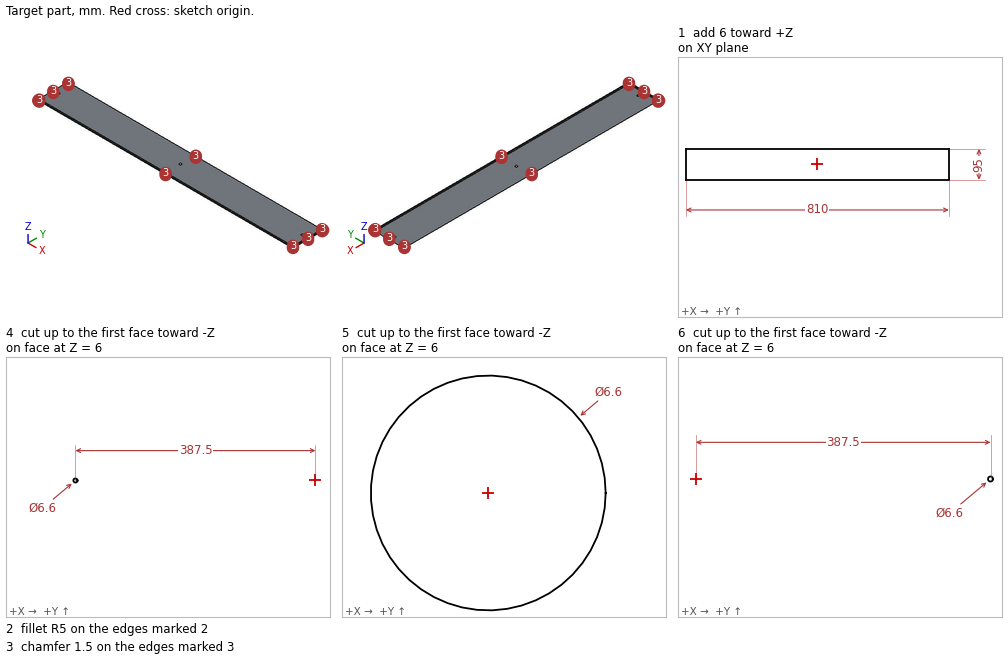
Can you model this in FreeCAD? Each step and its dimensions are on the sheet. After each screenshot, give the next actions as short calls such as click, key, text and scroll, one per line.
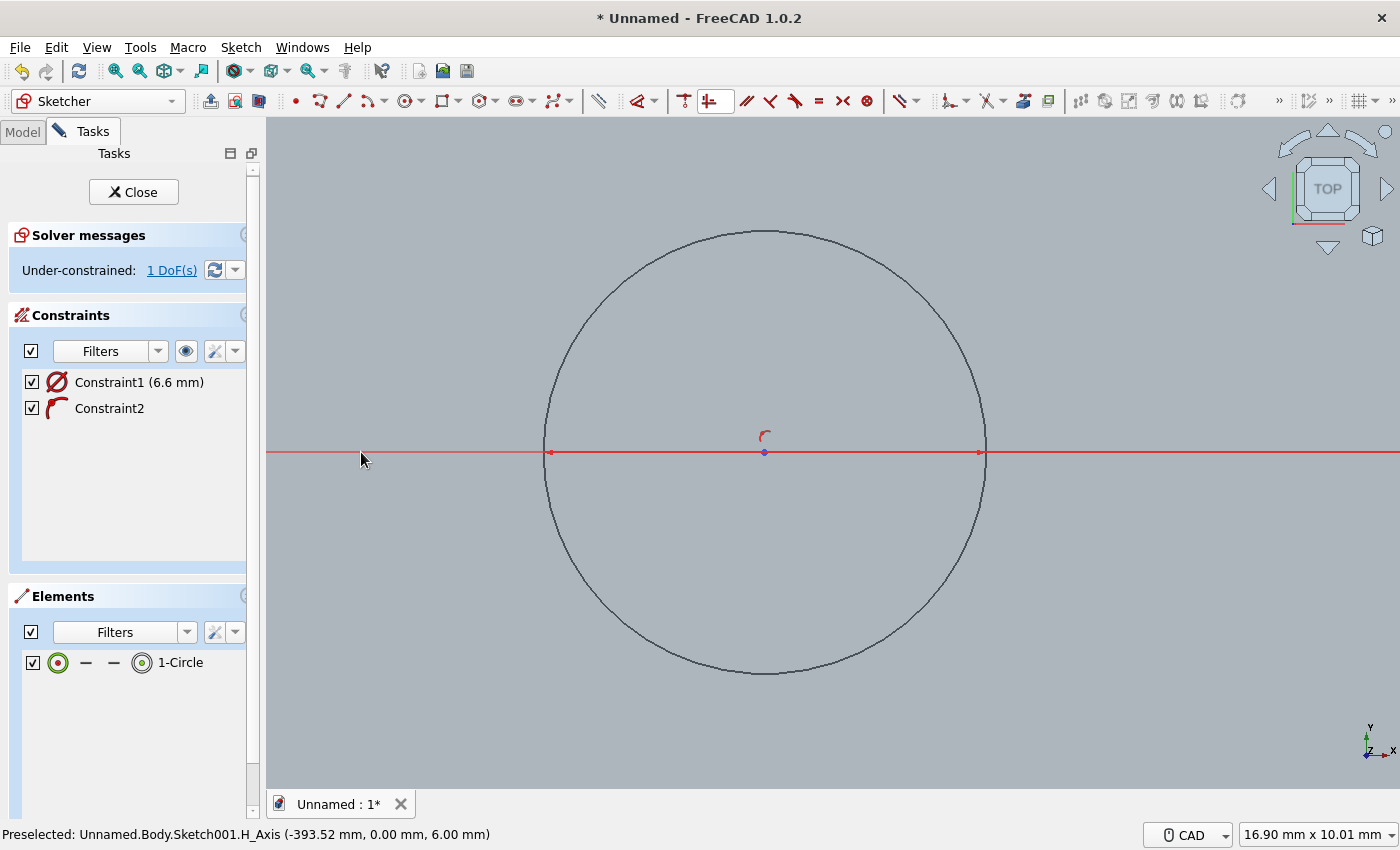
click(638, 102)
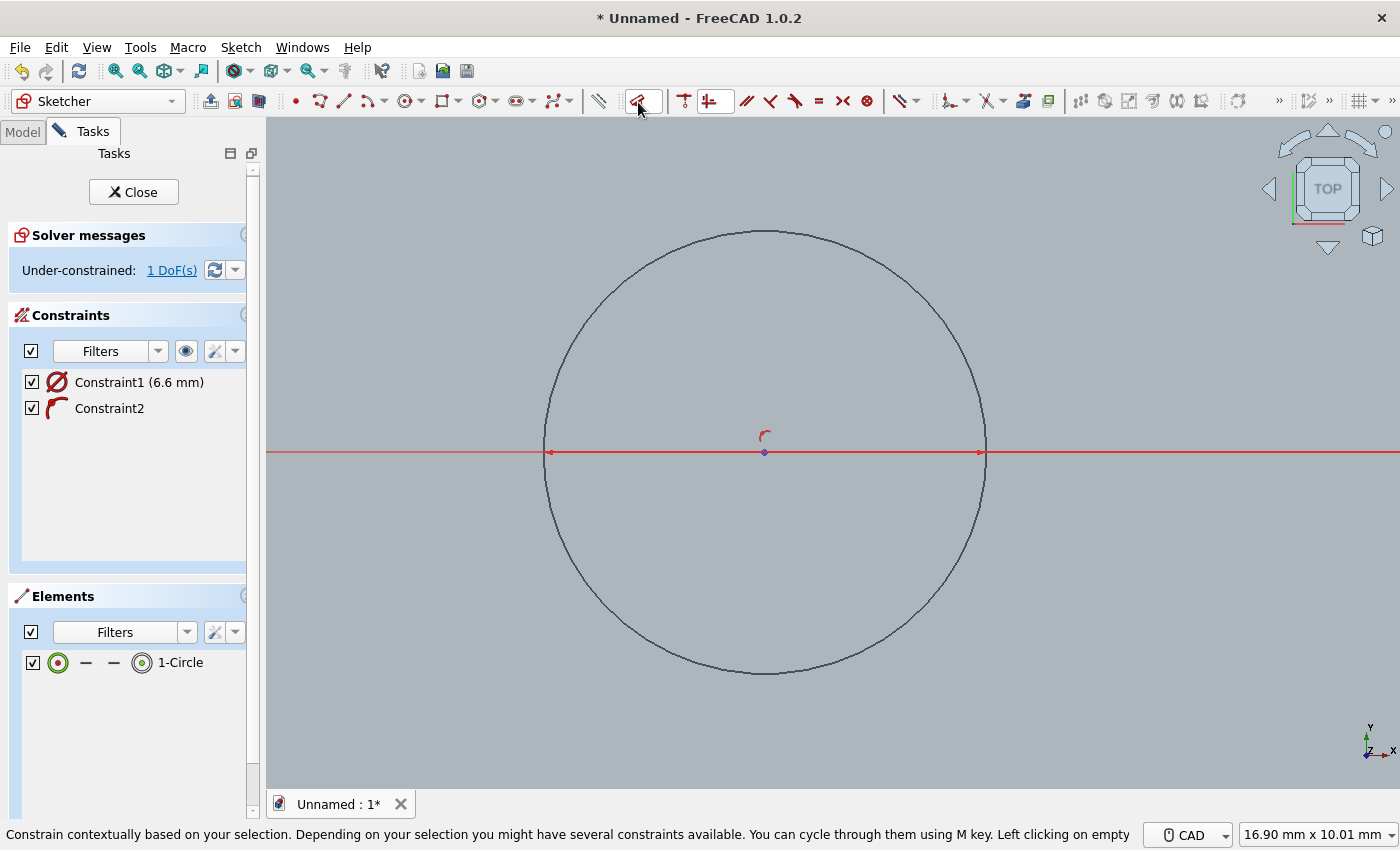
click(765, 452)
click(1000, 486)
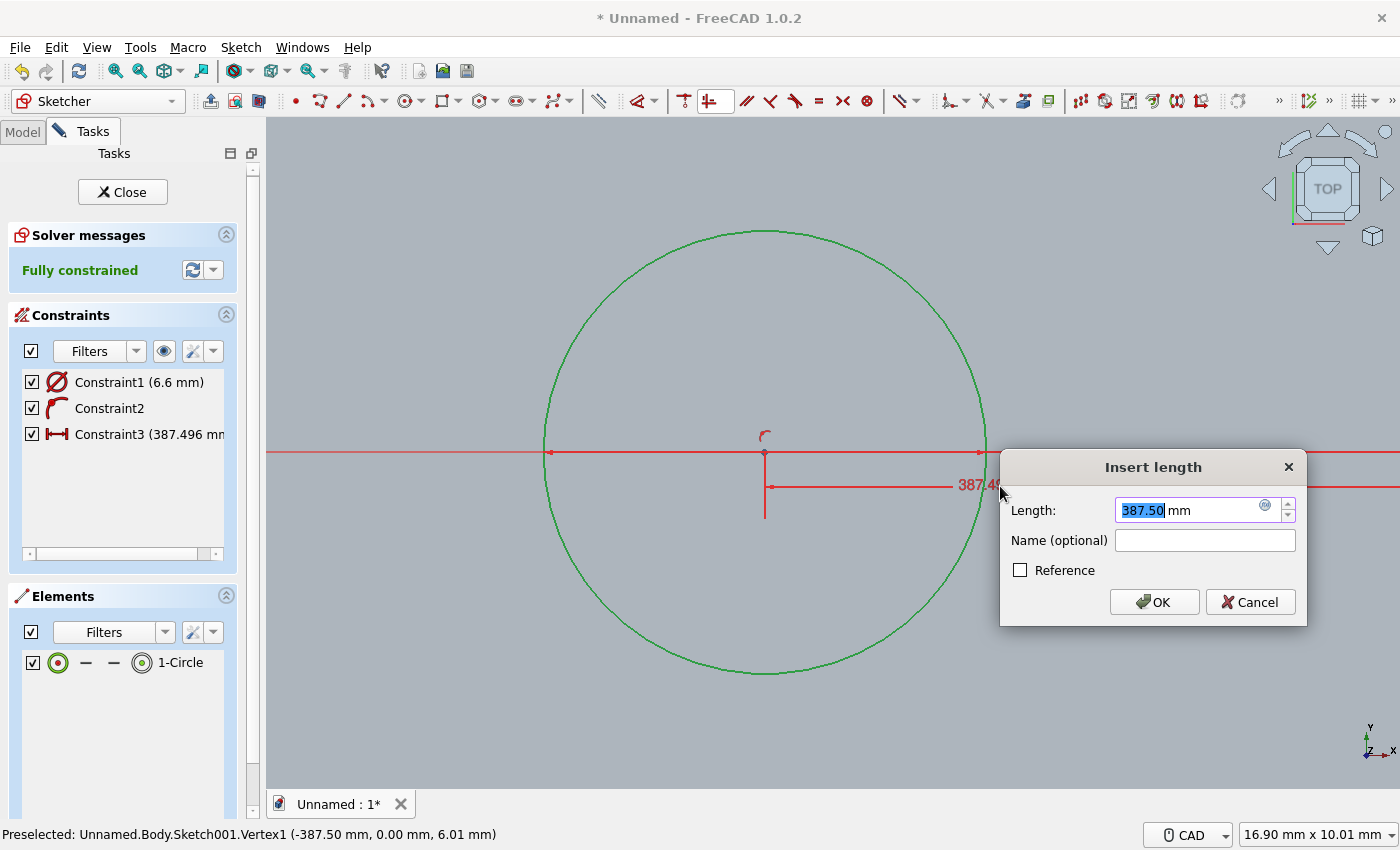
text(387.5)
key(Return)
key(Escape)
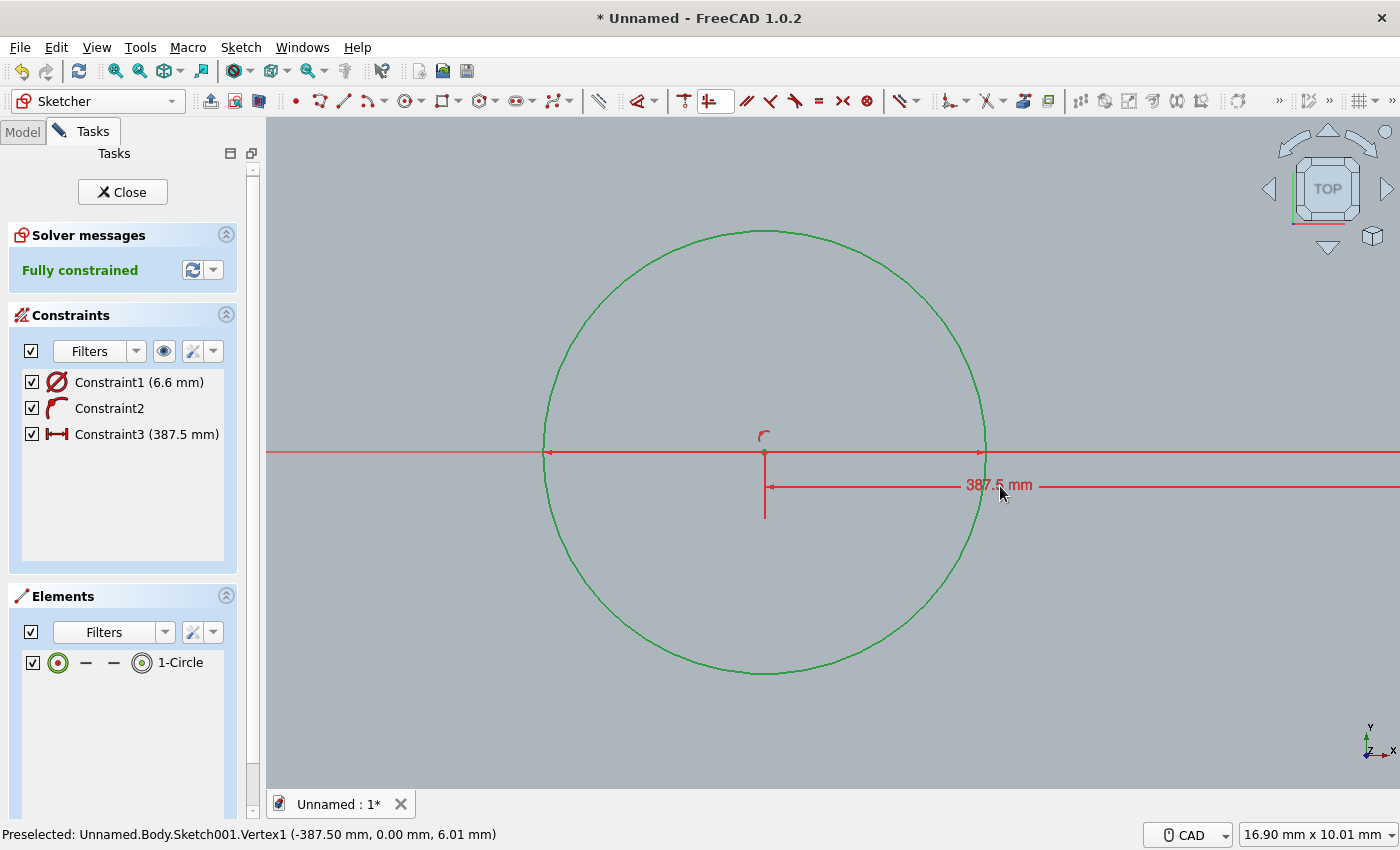
click(123, 192)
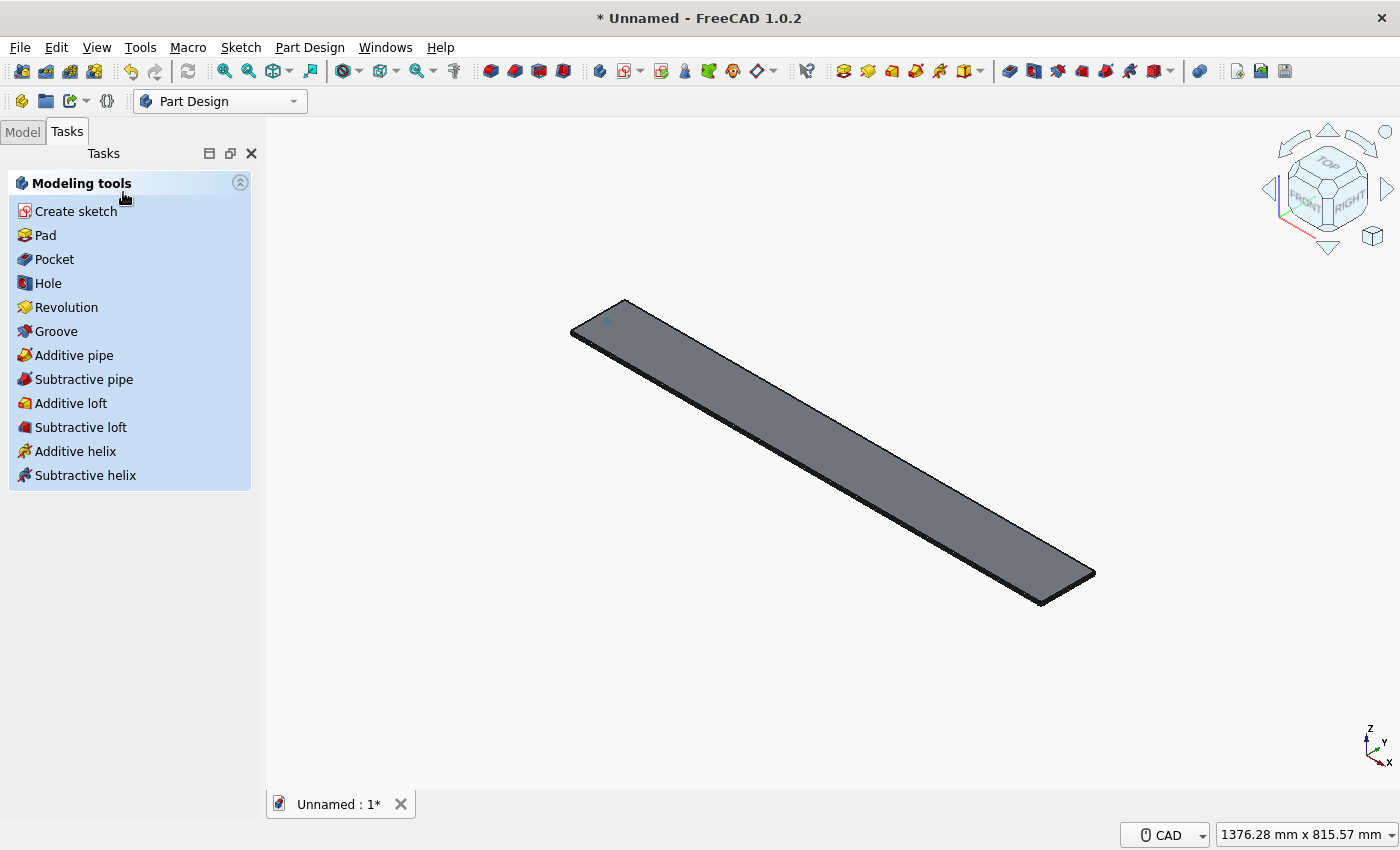
click(1010, 72)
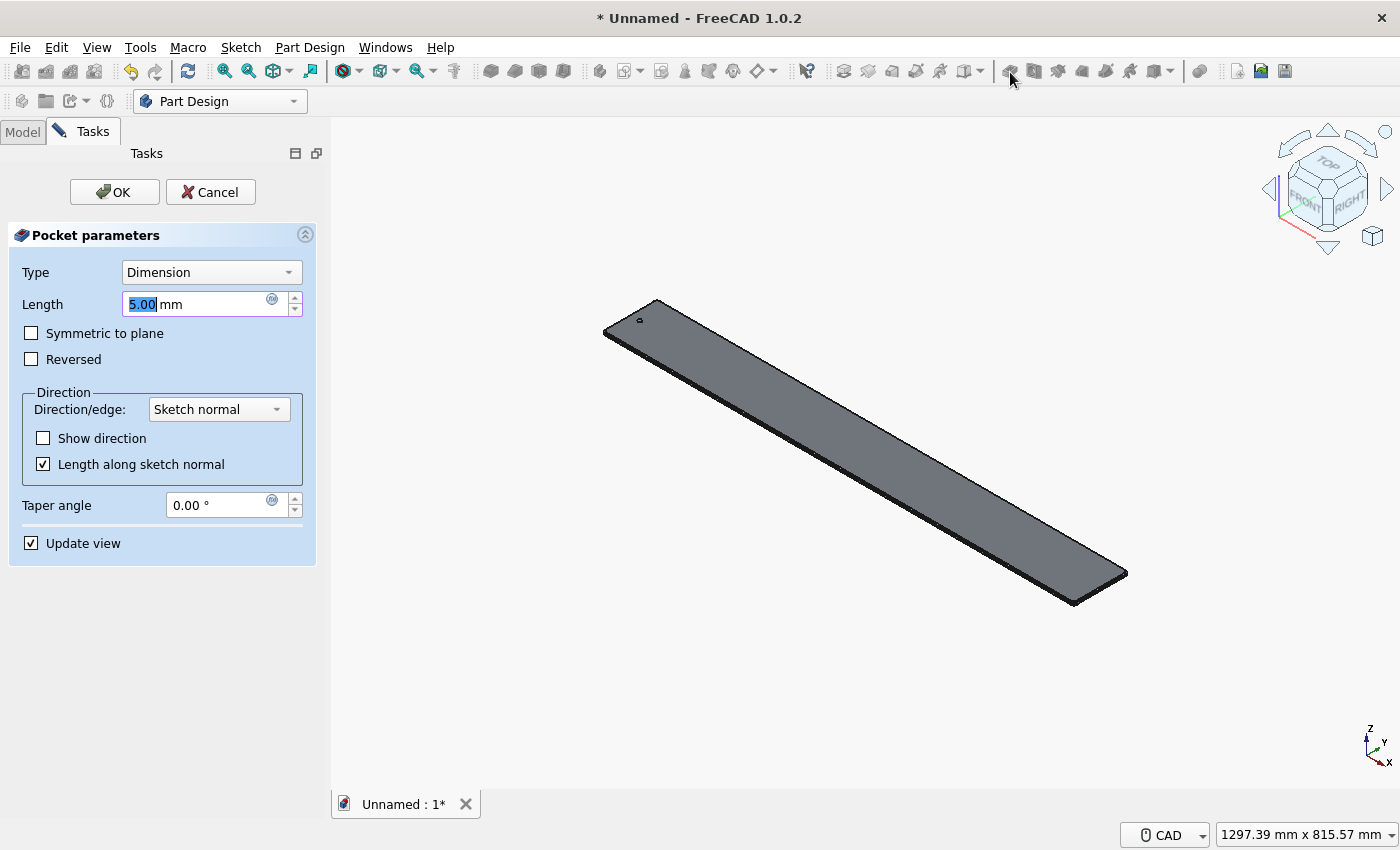
click(212, 272)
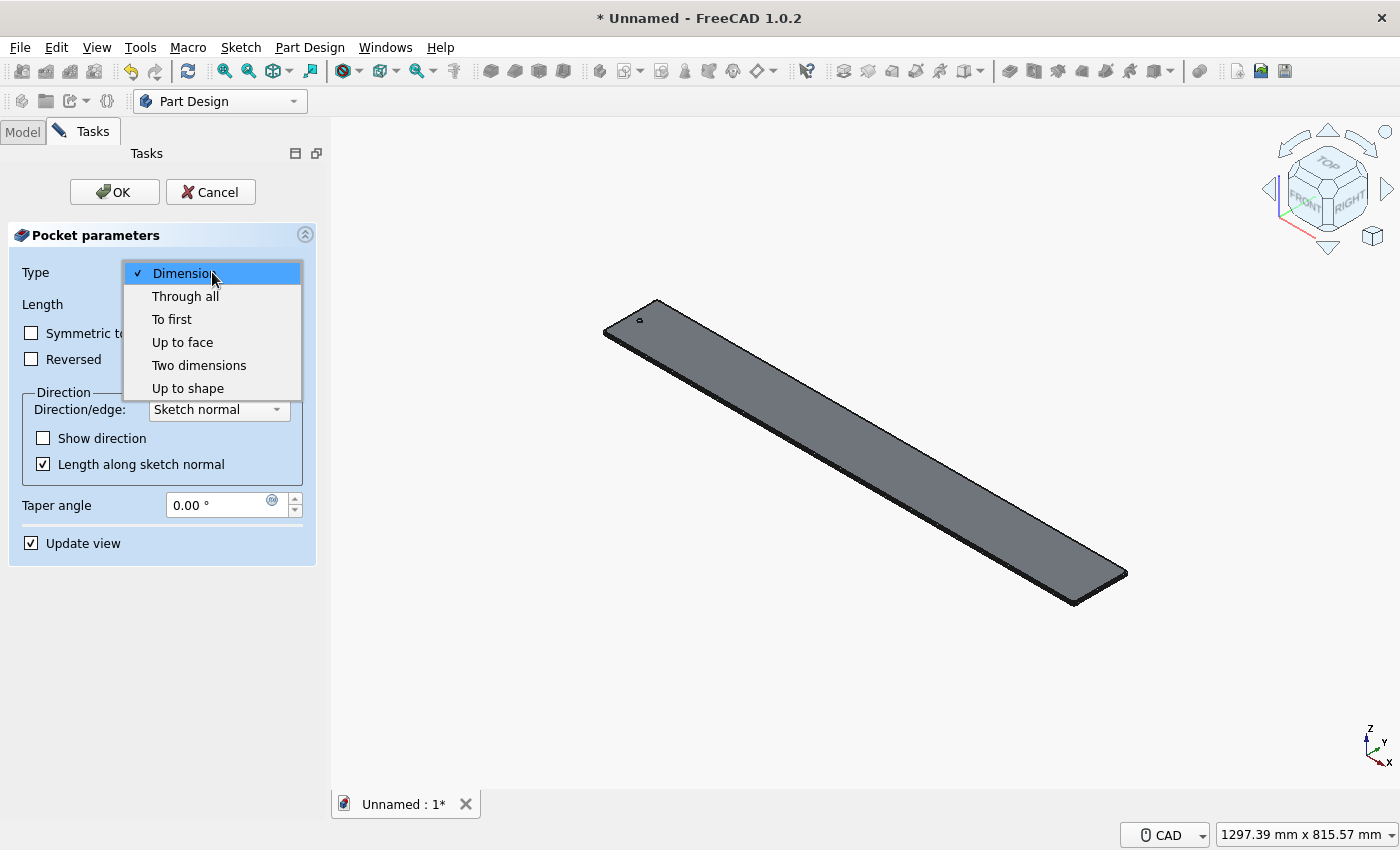
click(212, 320)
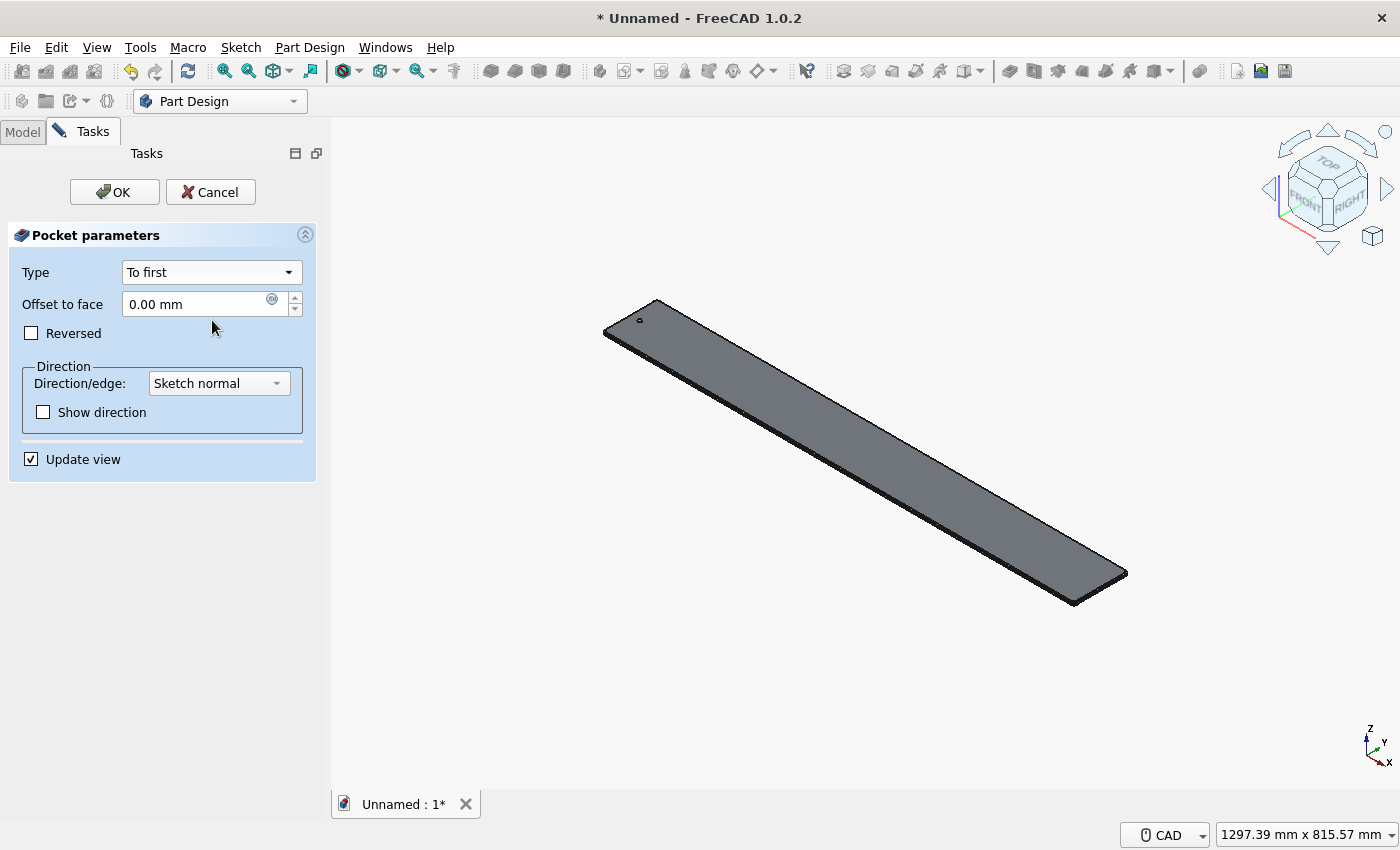
click(115, 192)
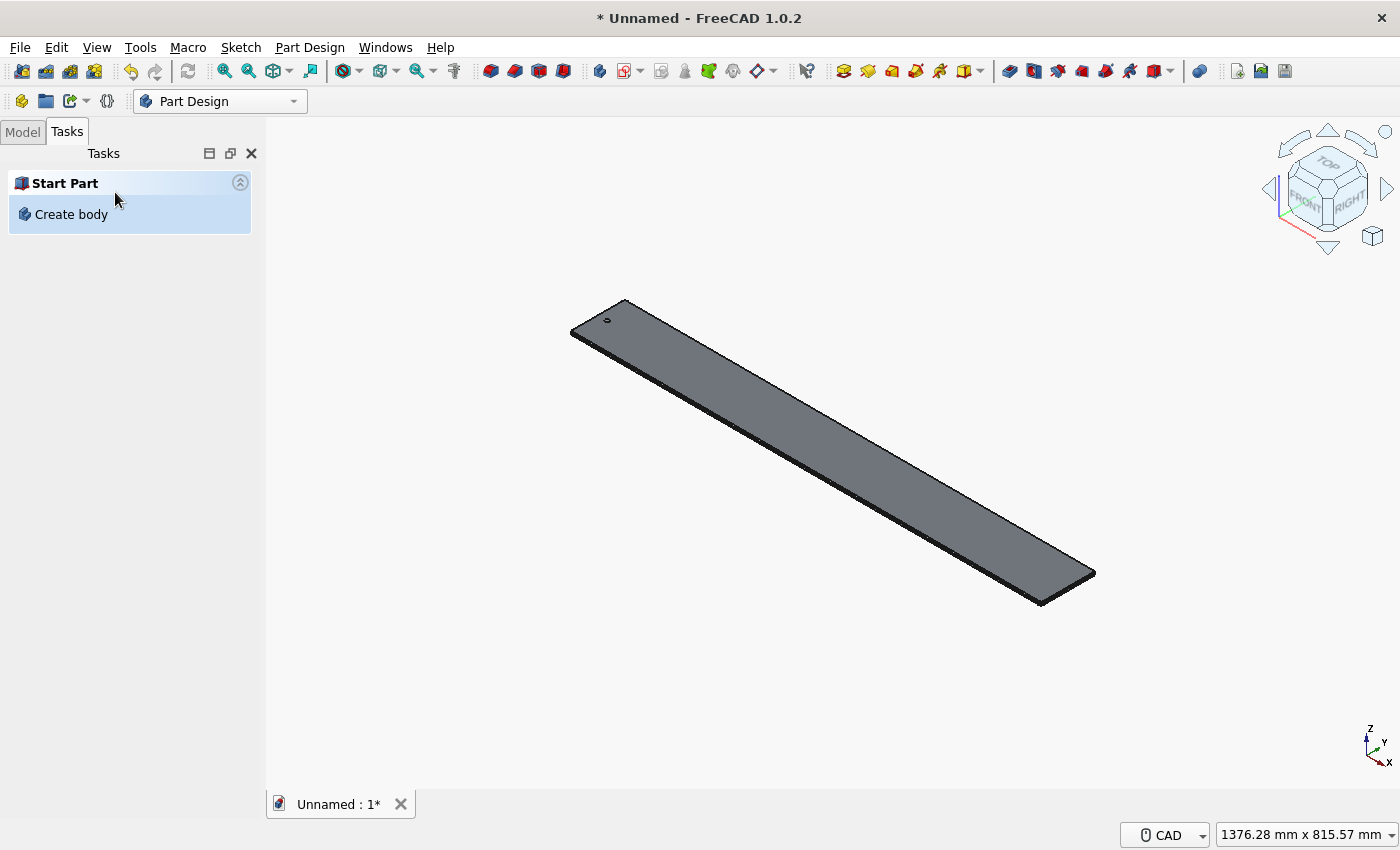
click(1035, 566)